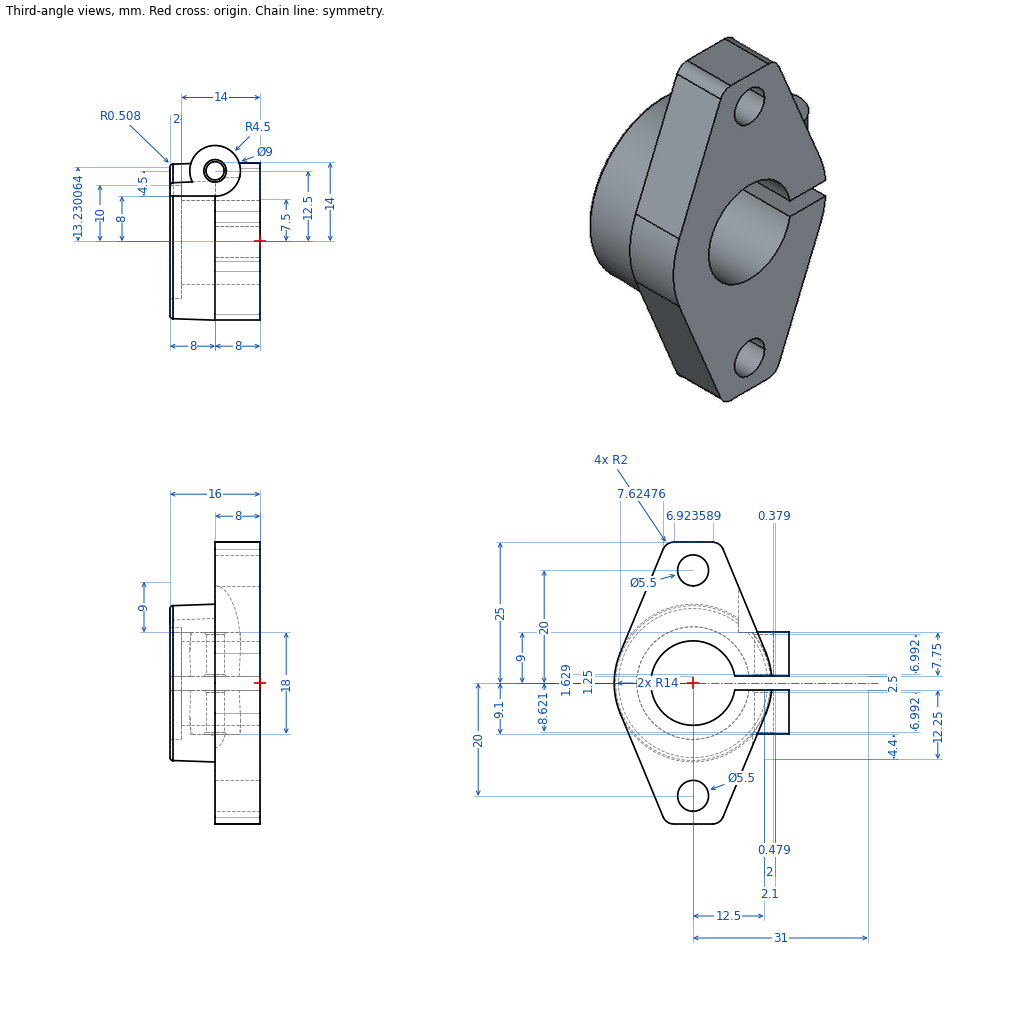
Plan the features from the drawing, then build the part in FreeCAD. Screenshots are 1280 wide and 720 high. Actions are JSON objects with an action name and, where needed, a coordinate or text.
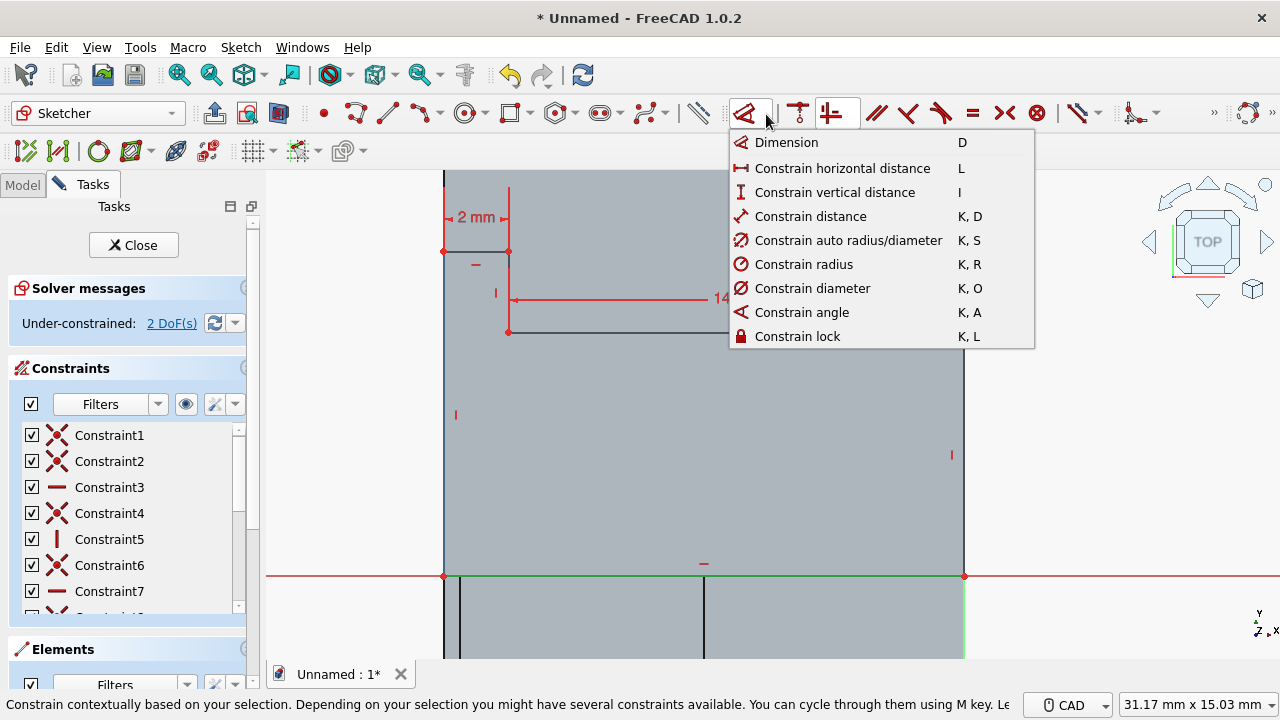
{"action": "left_click", "coordinate": [882, 192]}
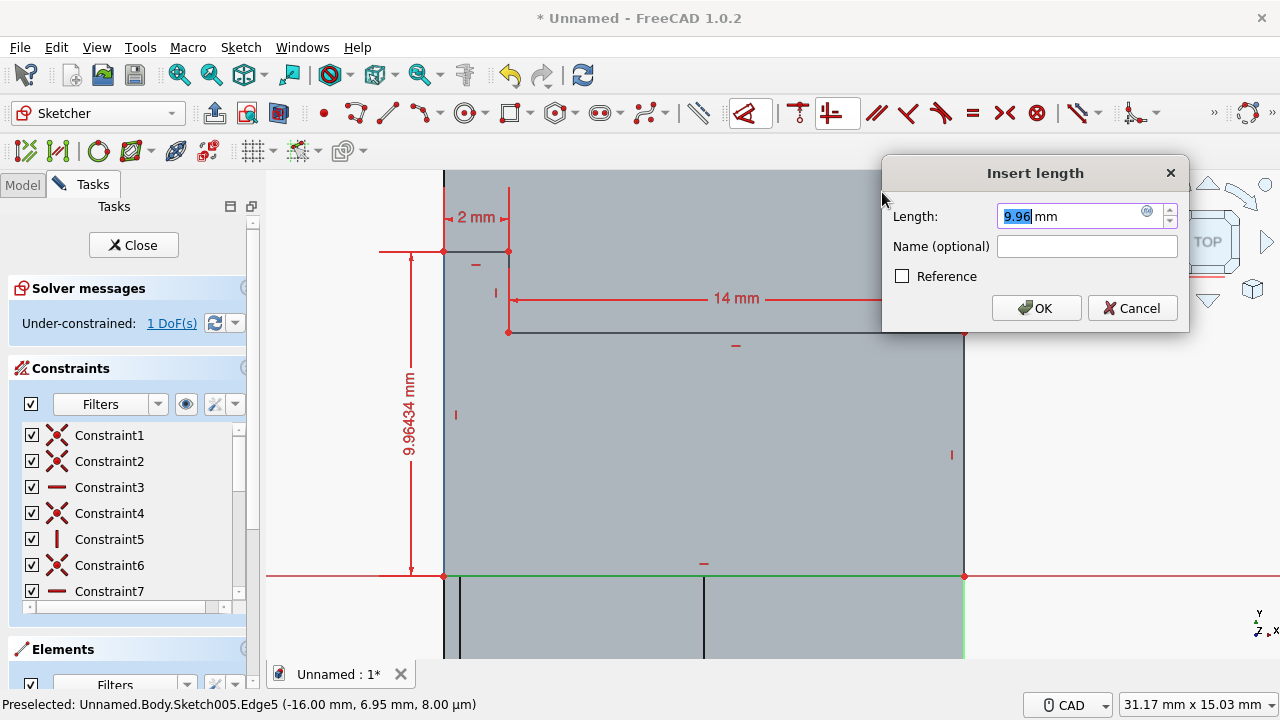
{"action": "type", "text": "10"}
{"action": "key", "text": "Return"}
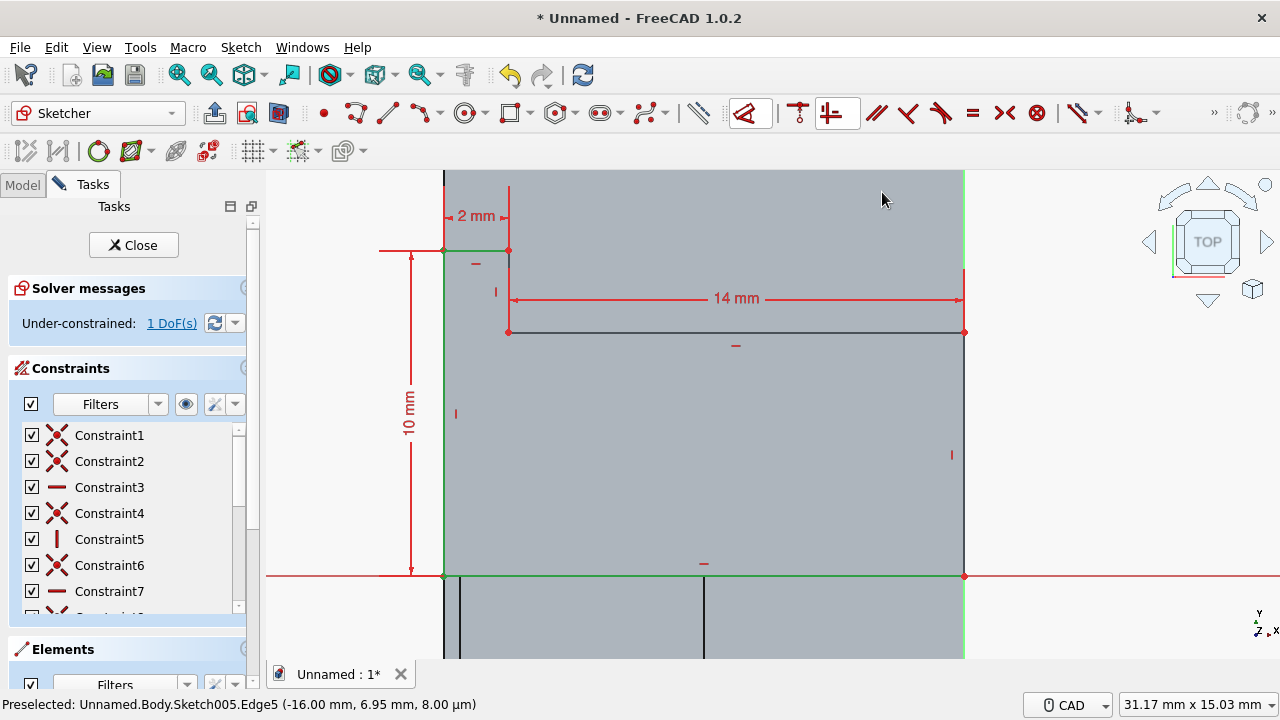
{"action": "left_click", "coordinate": [964, 503]}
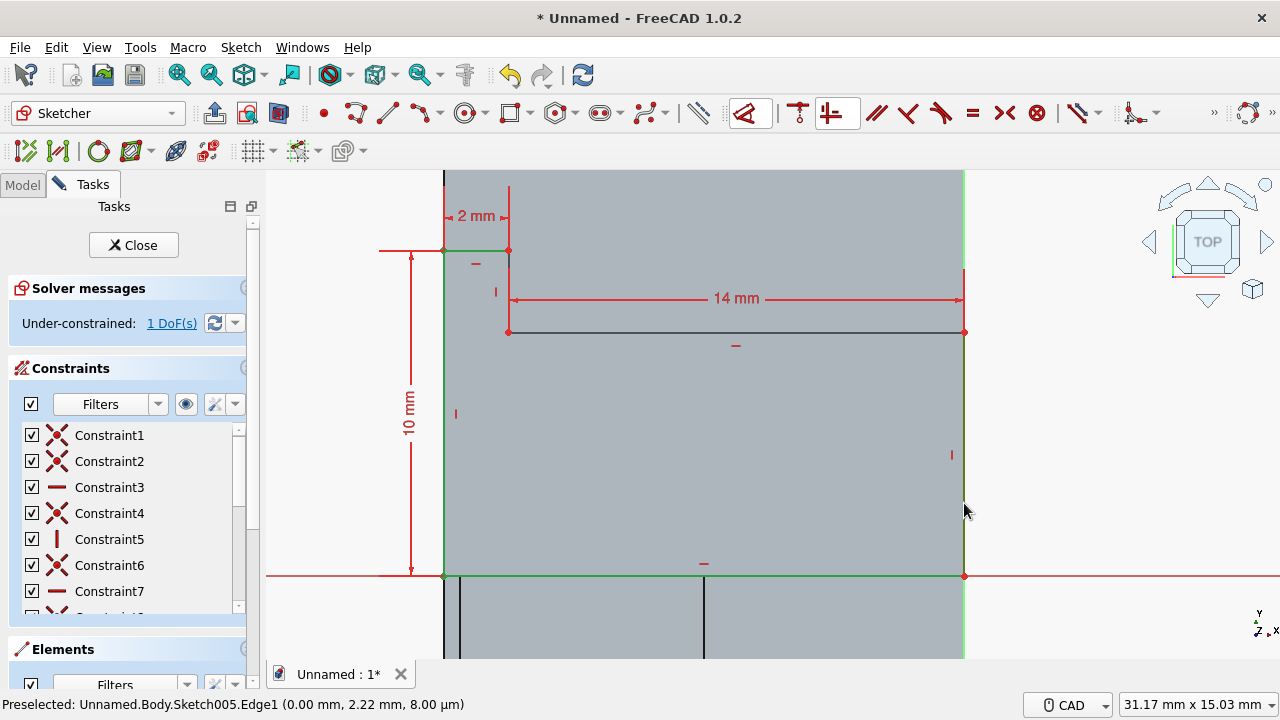
{"action": "key", "text": "i"}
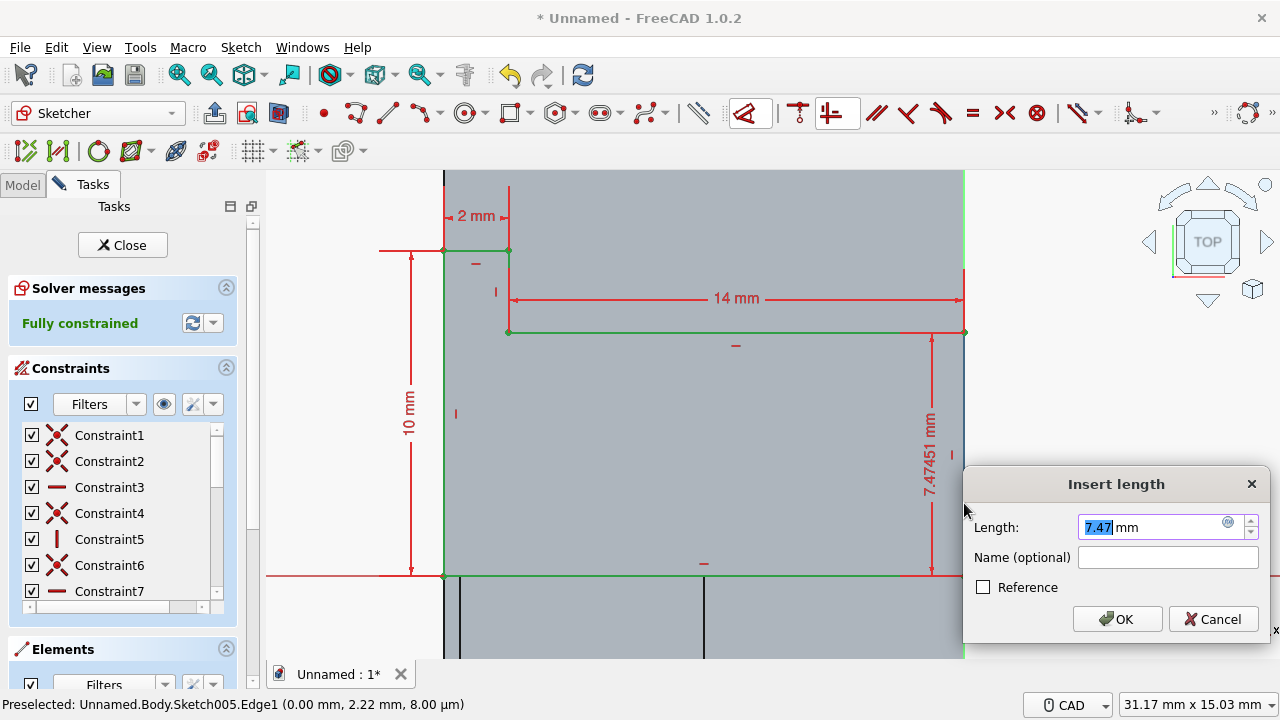
{"action": "type", "text": "7.5"}
{"action": "key", "text": "Return"}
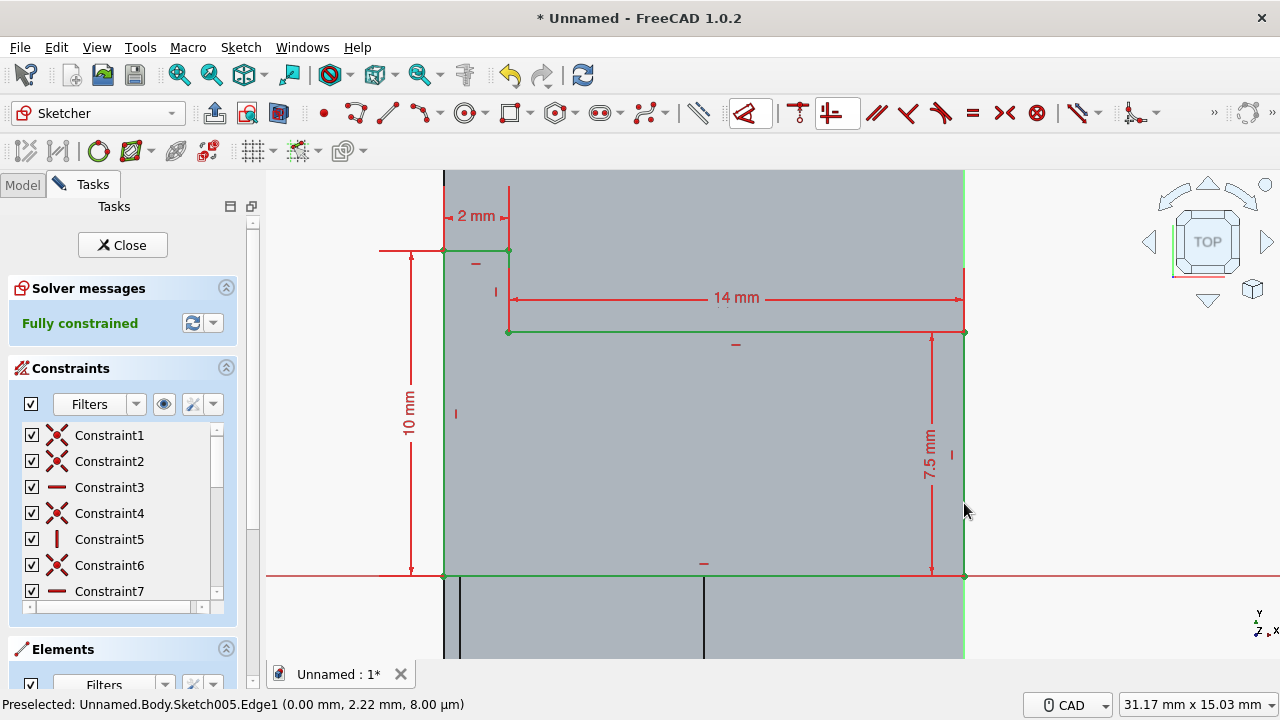
{"action": "left_click", "coordinate": [123, 245]}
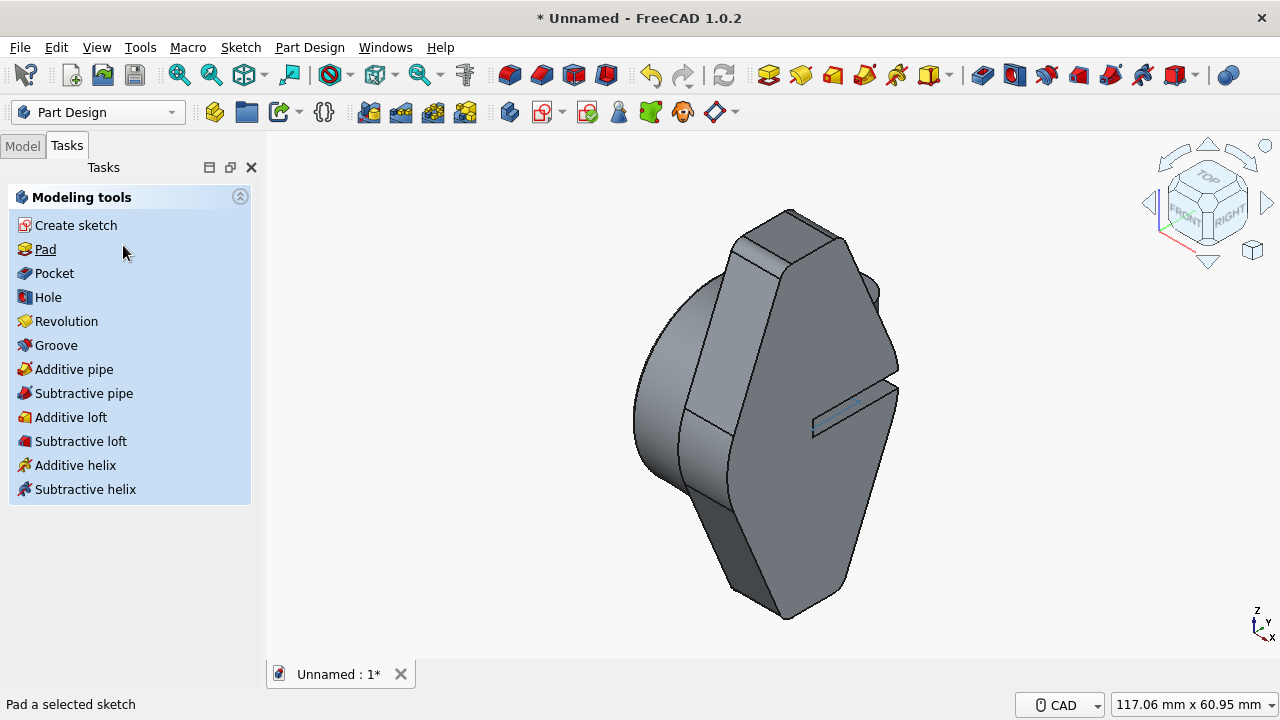
{"action": "left_click", "coordinate": [1048, 76]}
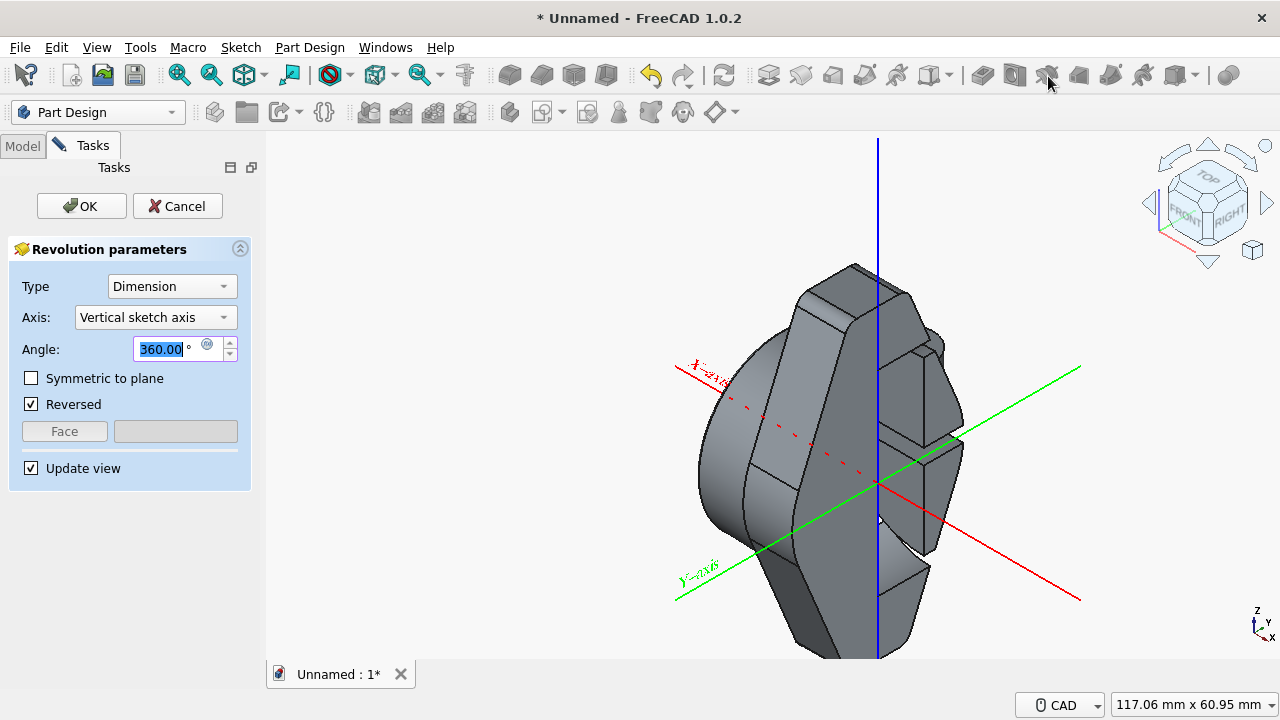
{"action": "left_click", "coordinate": [156, 318]}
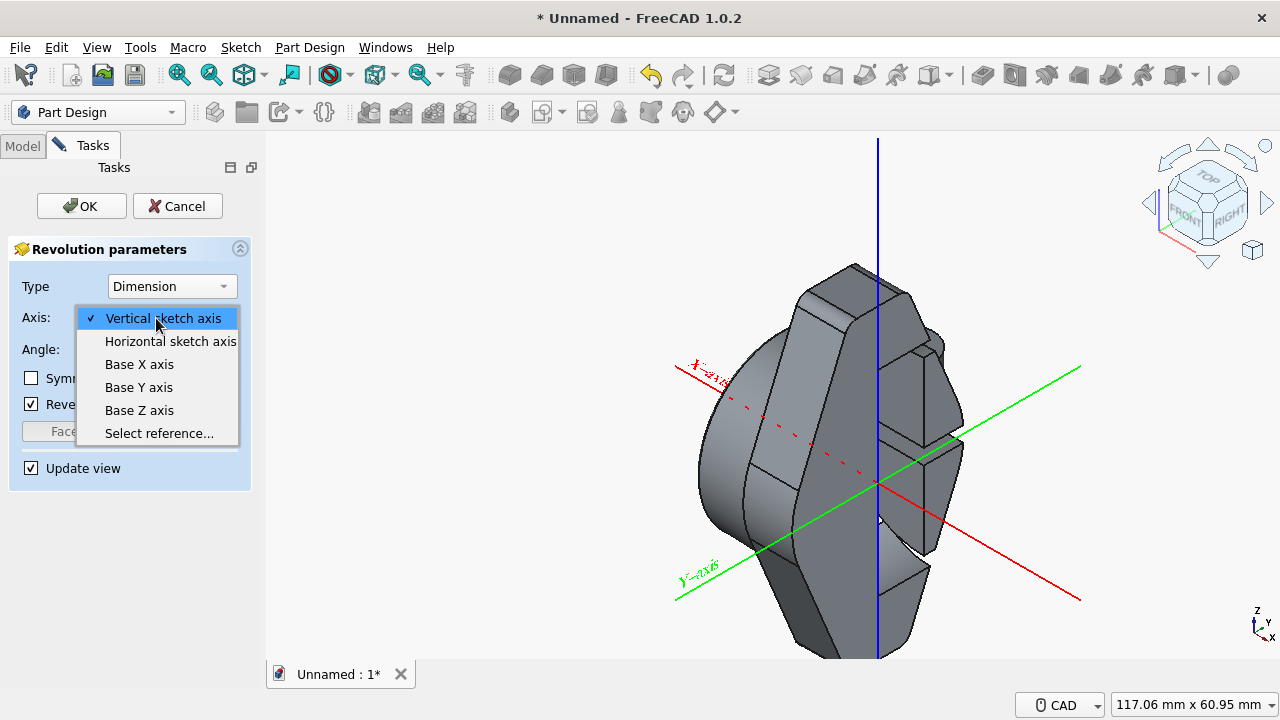
{"action": "left_click", "coordinate": [156, 342]}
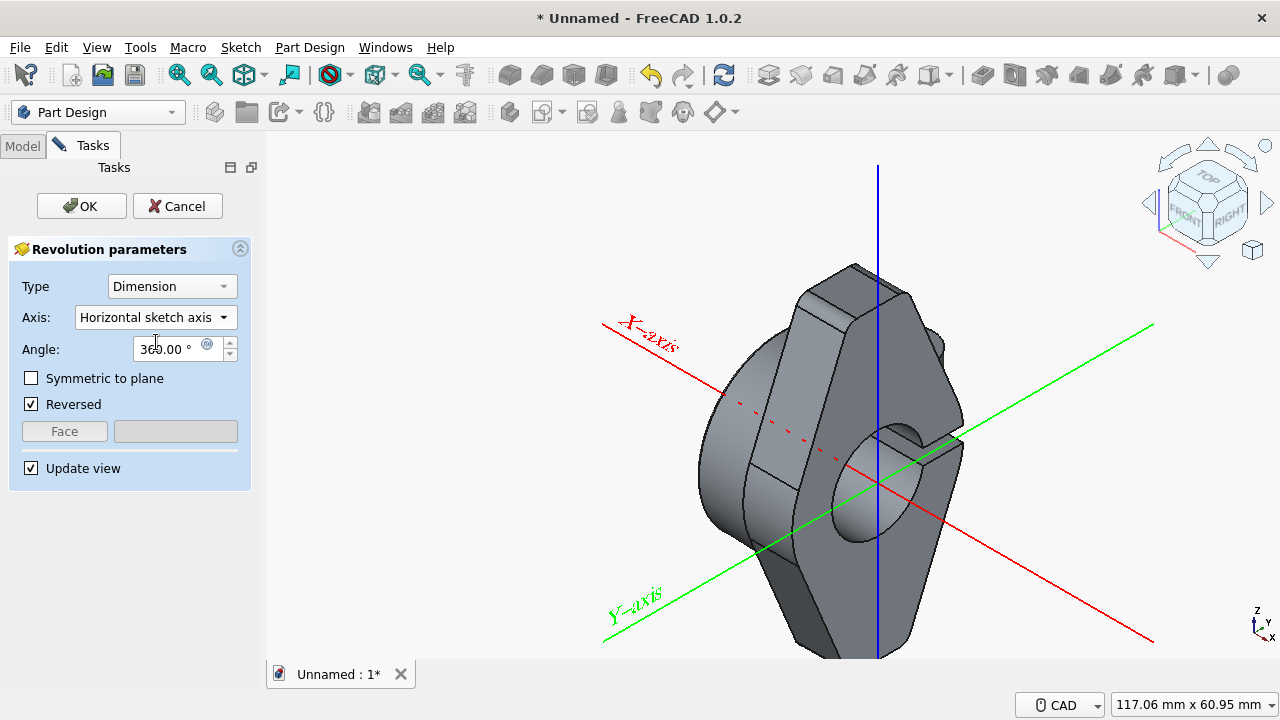
{"action": "left_click", "coordinate": [82, 206]}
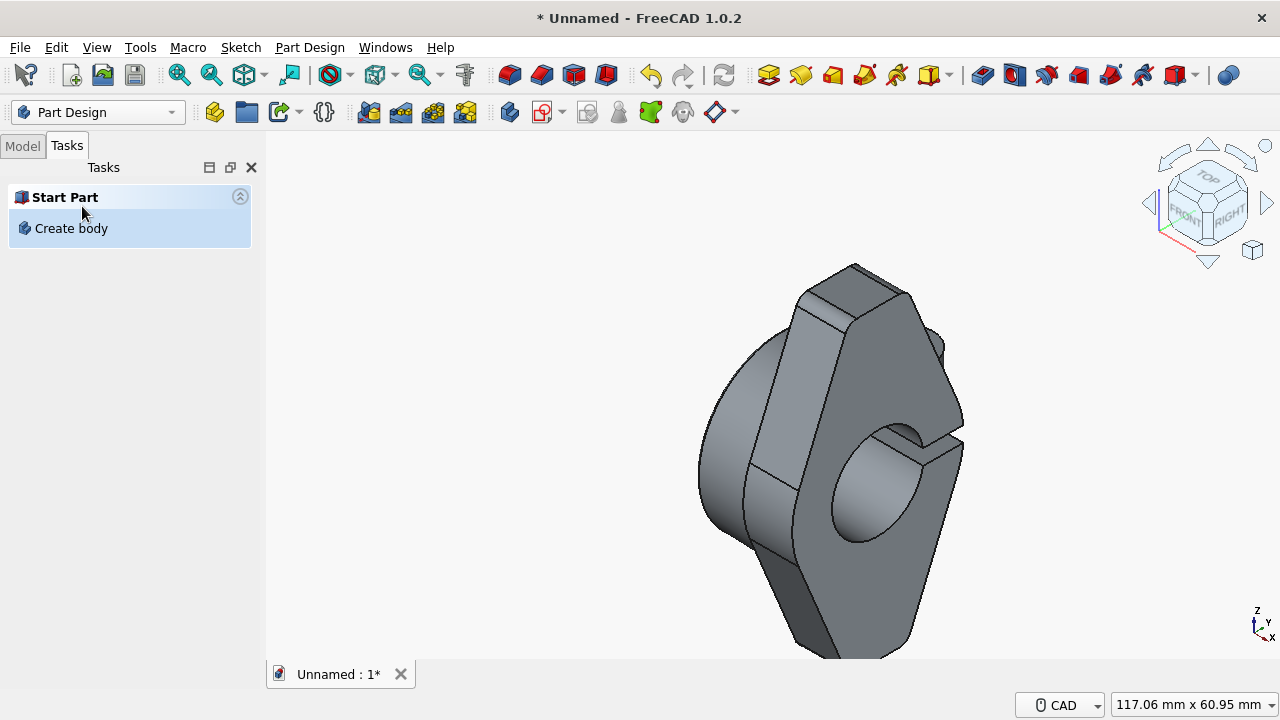
{"action": "key", "text": "v f"}